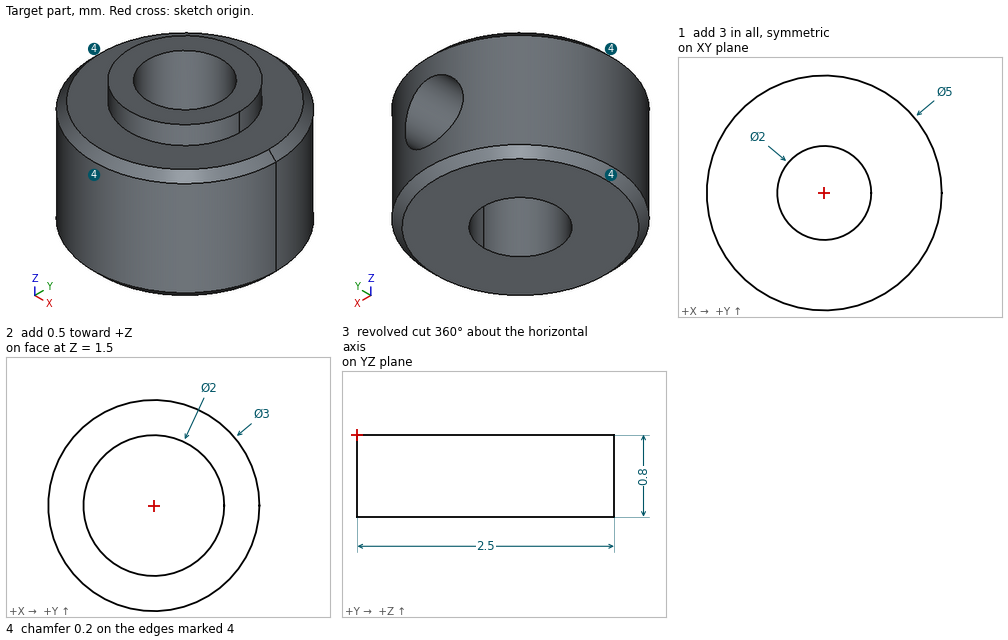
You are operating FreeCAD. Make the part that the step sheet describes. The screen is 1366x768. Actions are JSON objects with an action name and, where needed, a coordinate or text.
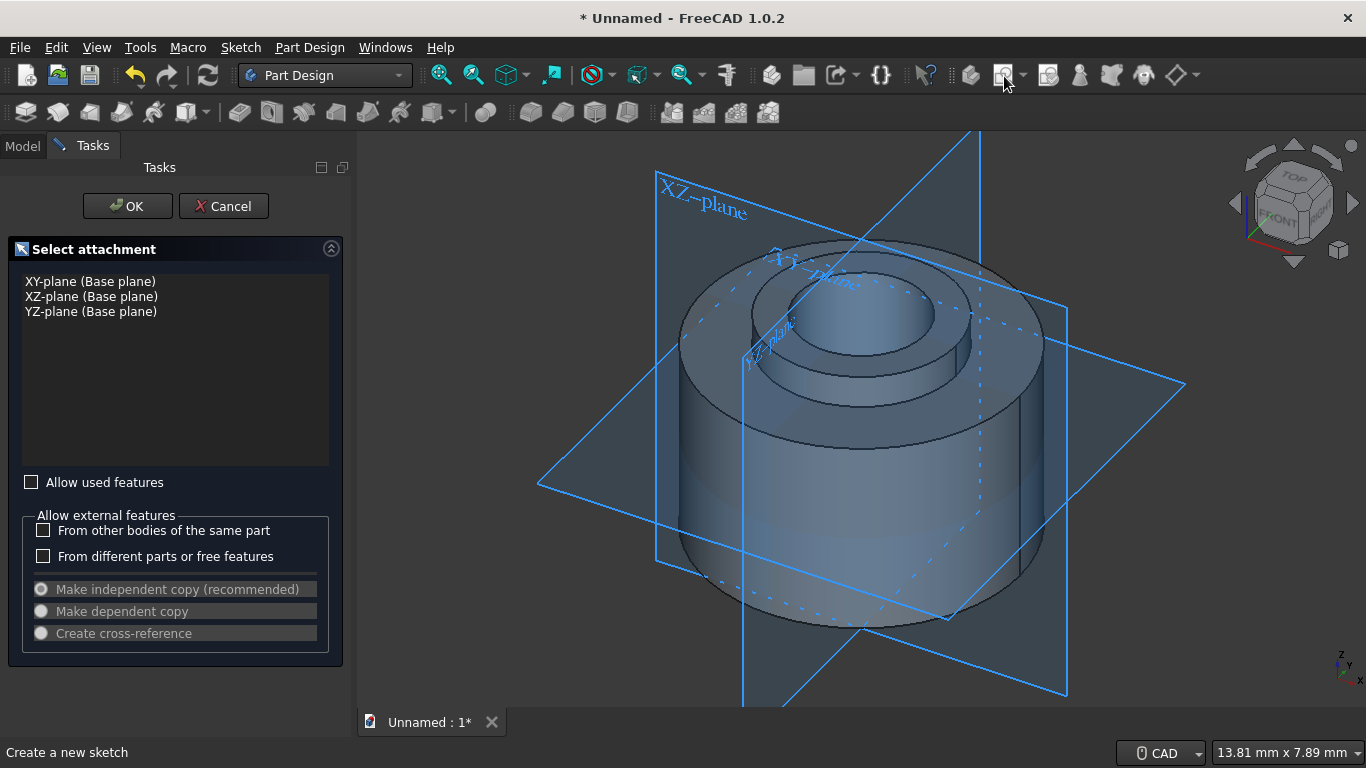
{"action": "left_click", "coordinate": [82, 312]}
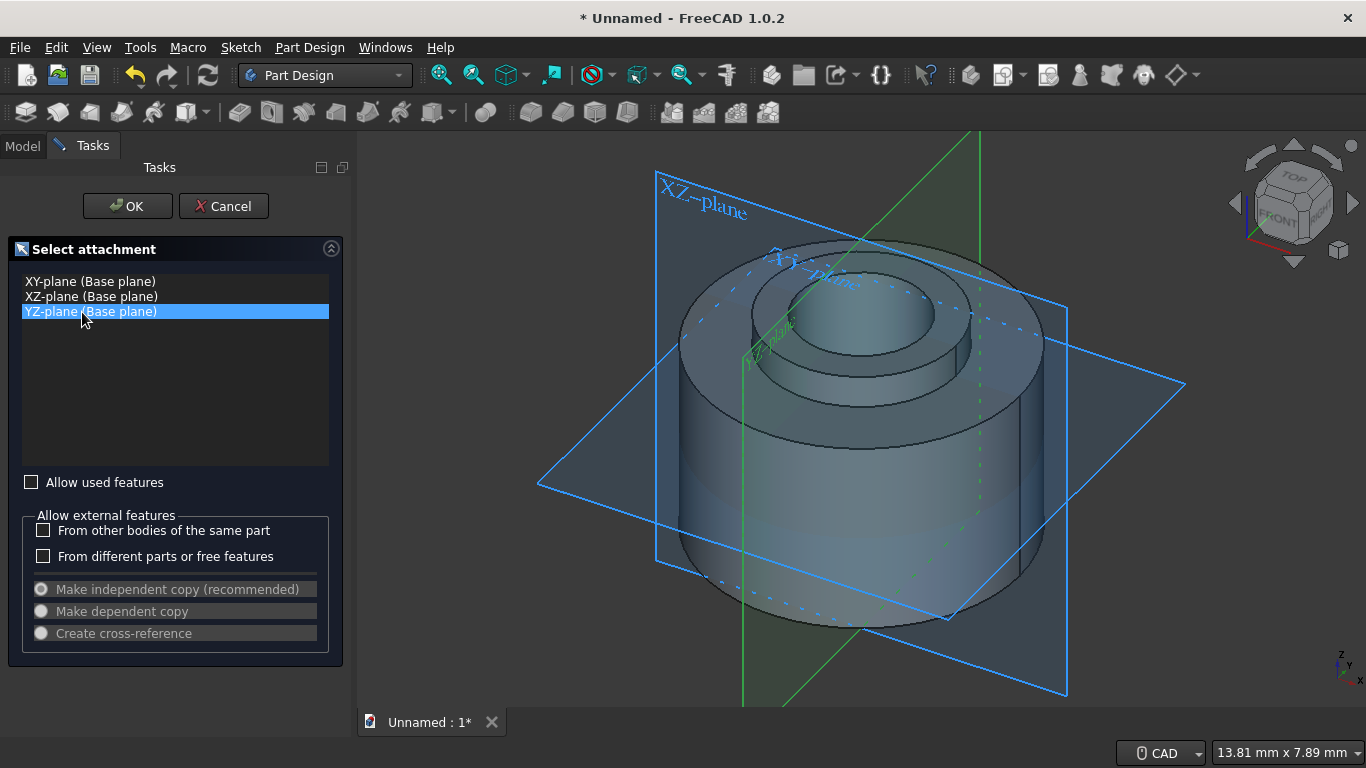
{"action": "left_click", "coordinate": [128, 206]}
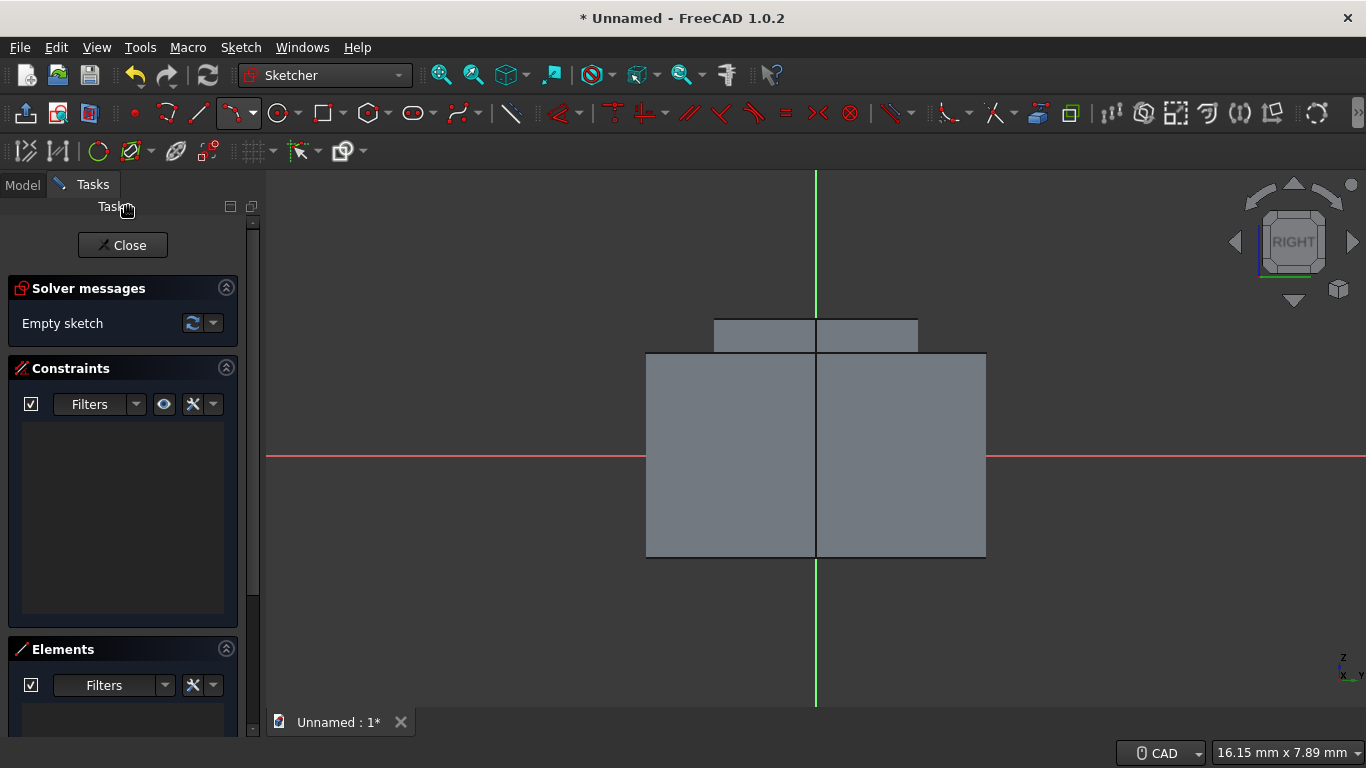
{"action": "key", "text": "q s"}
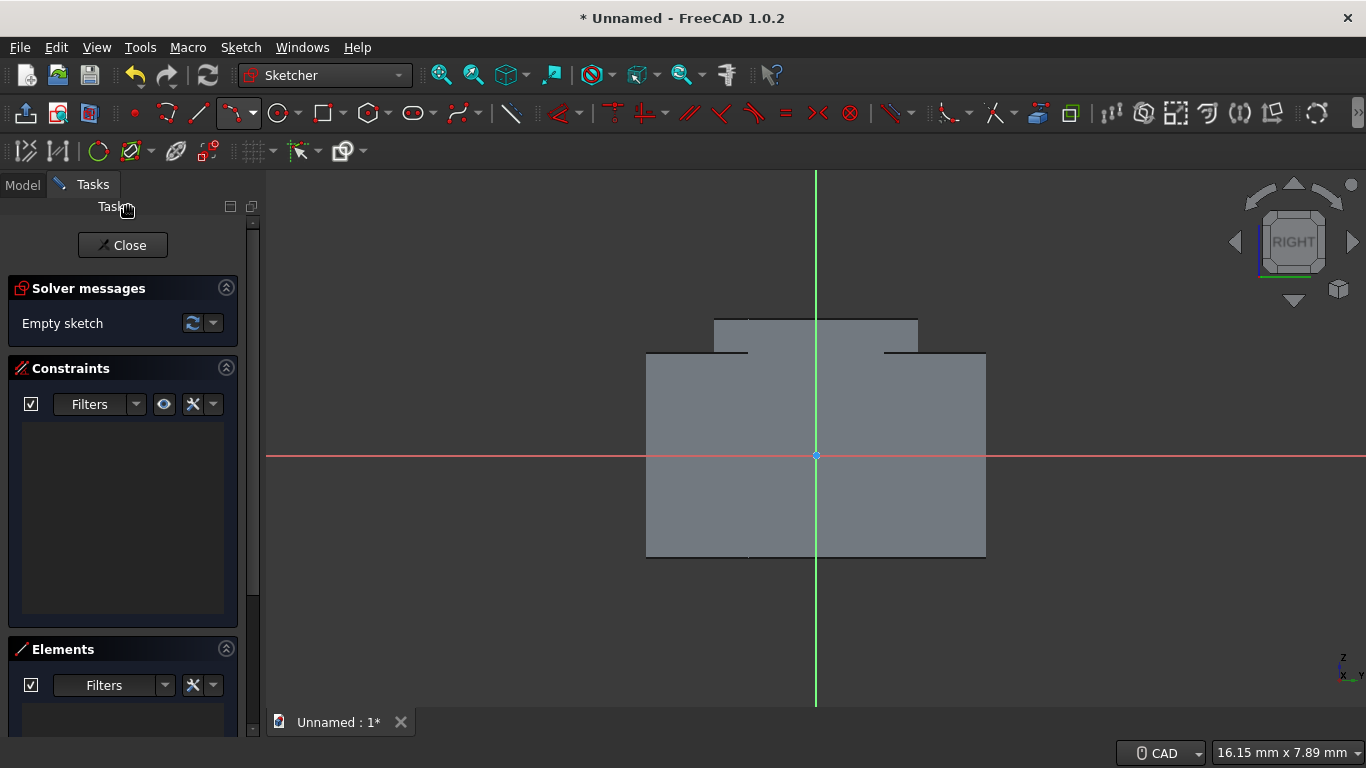
{"action": "scroll", "coordinate": [951, 497], "scroll_direction": "up", "scroll_amount": 7}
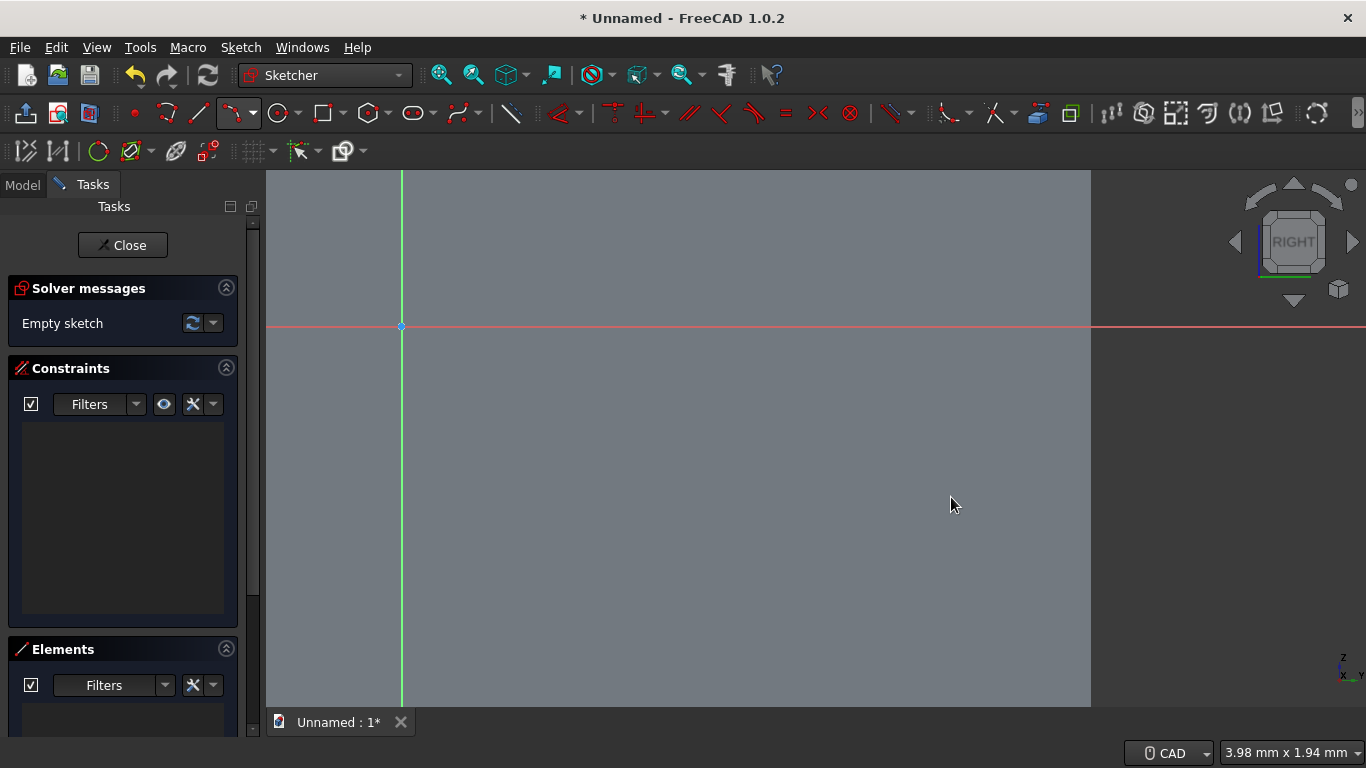
{"action": "left_click", "coordinate": [324, 114]}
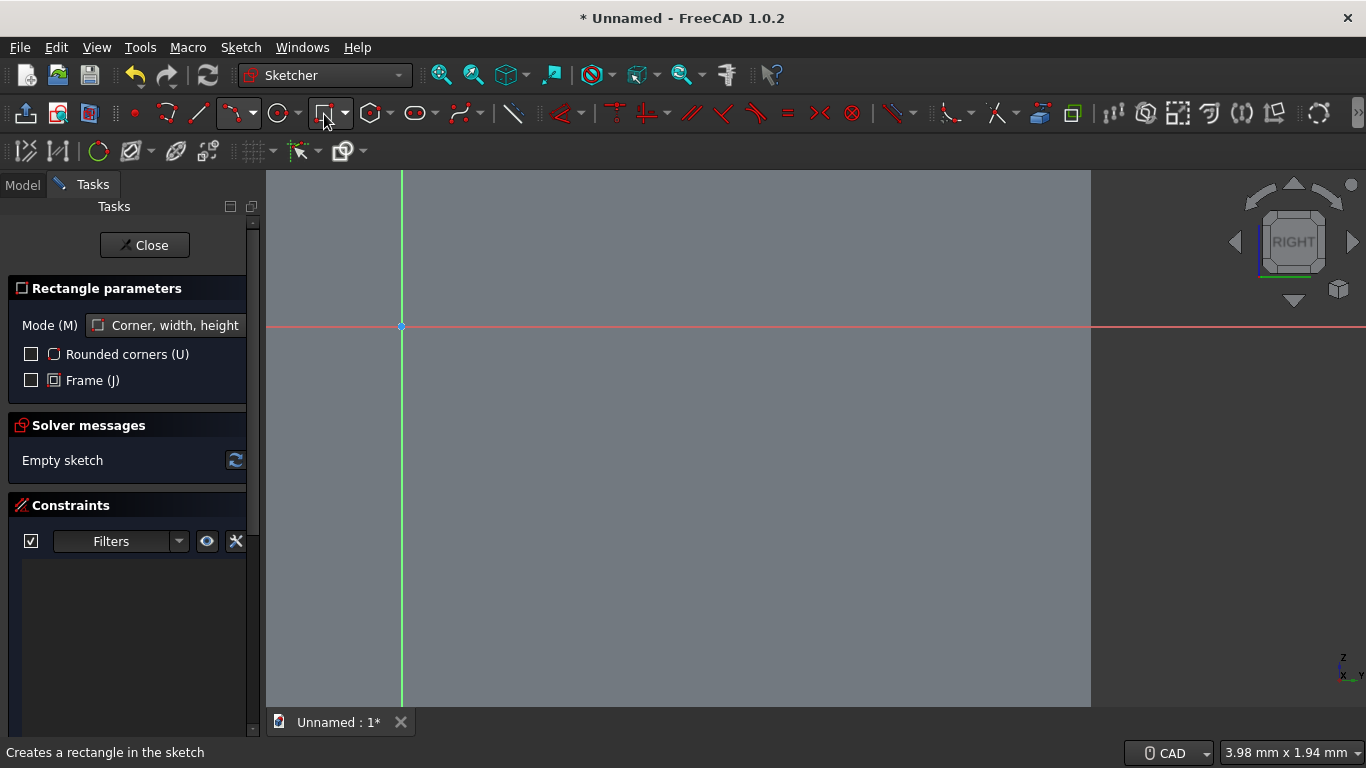
{"action": "left_click", "coordinate": [402, 327]}
{"action": "mouse_move", "coordinate": [1092, 548]}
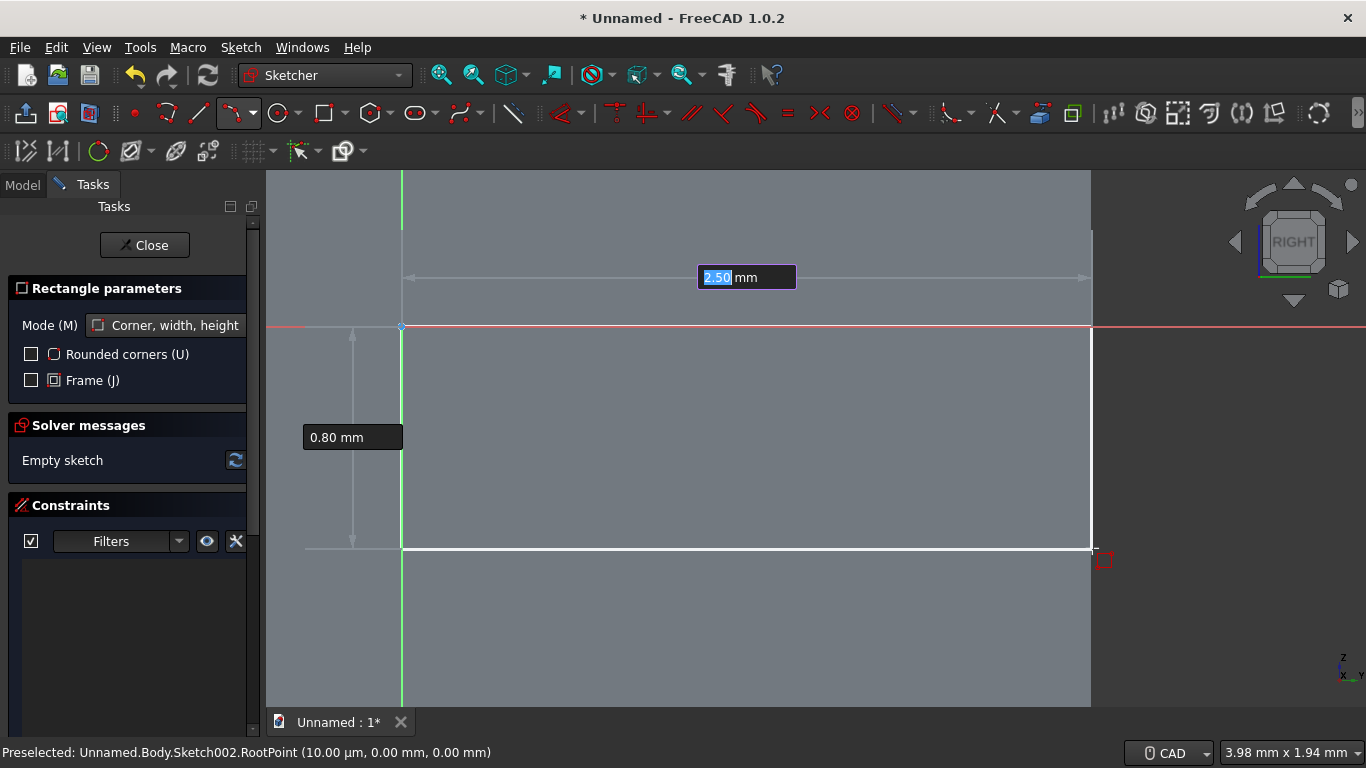
{"action": "type", "text": "2.5"}
{"action": "key", "text": "Tab"}
{"action": "type", "text": "0.8"}
{"action": "key", "text": "Return"}
{"action": "key", "text": "Escape"}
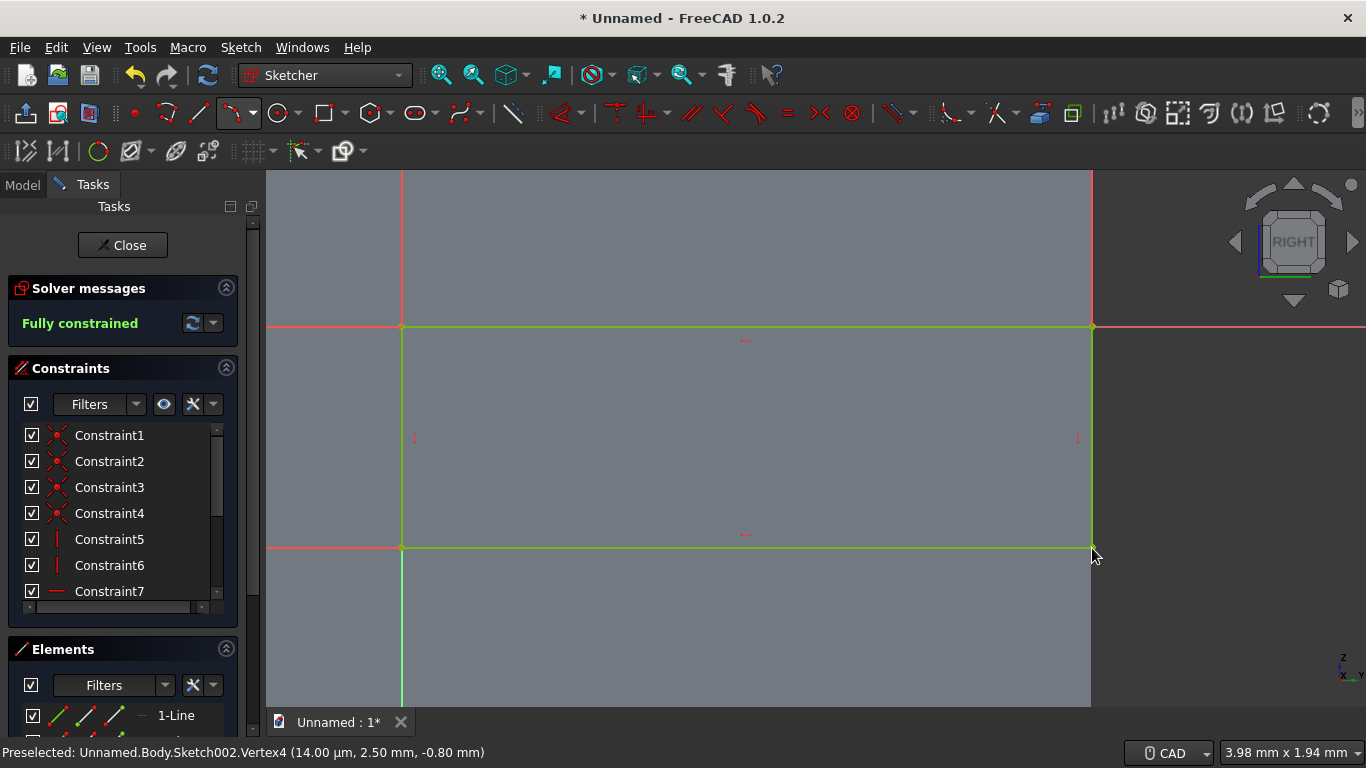
{"action": "left_click", "coordinate": [123, 245]}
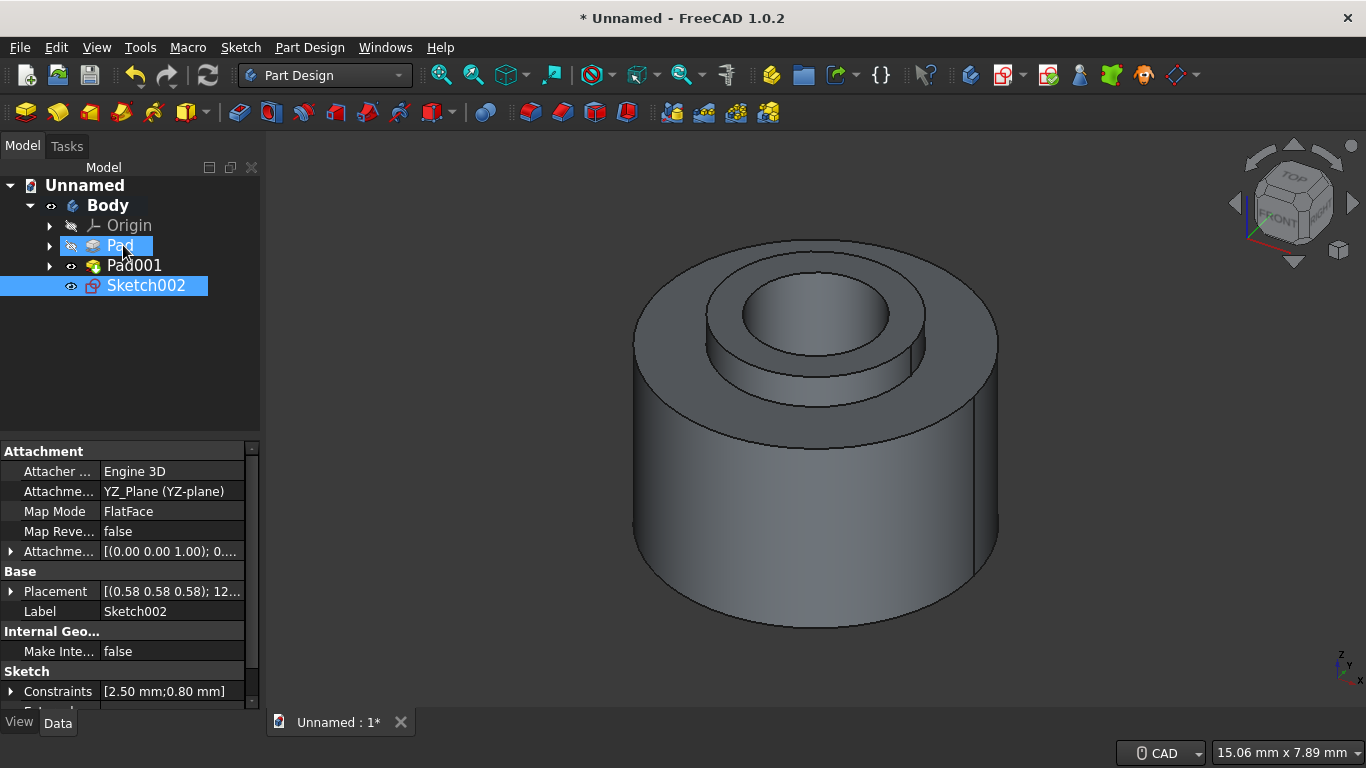
{"action": "left_click", "coordinate": [304, 112]}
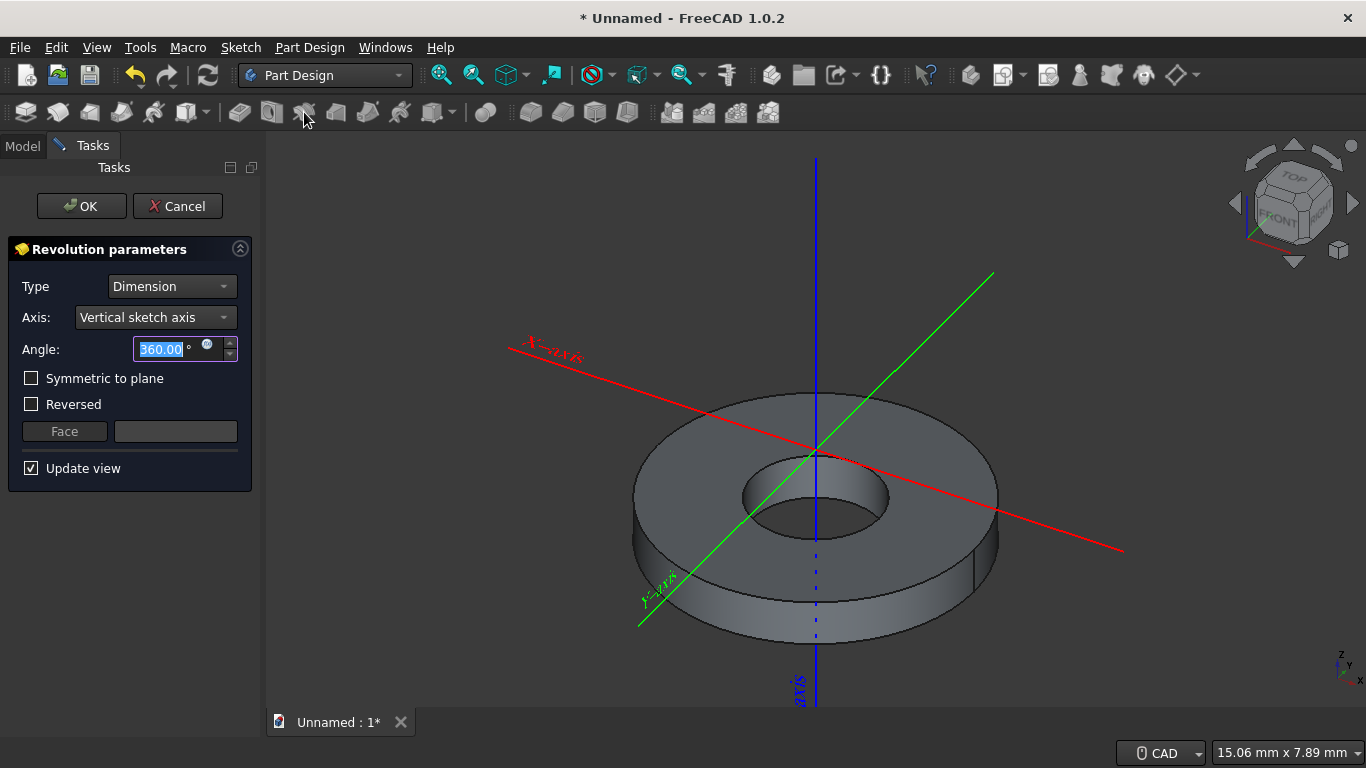
{"action": "left_click", "coordinate": [156, 318]}